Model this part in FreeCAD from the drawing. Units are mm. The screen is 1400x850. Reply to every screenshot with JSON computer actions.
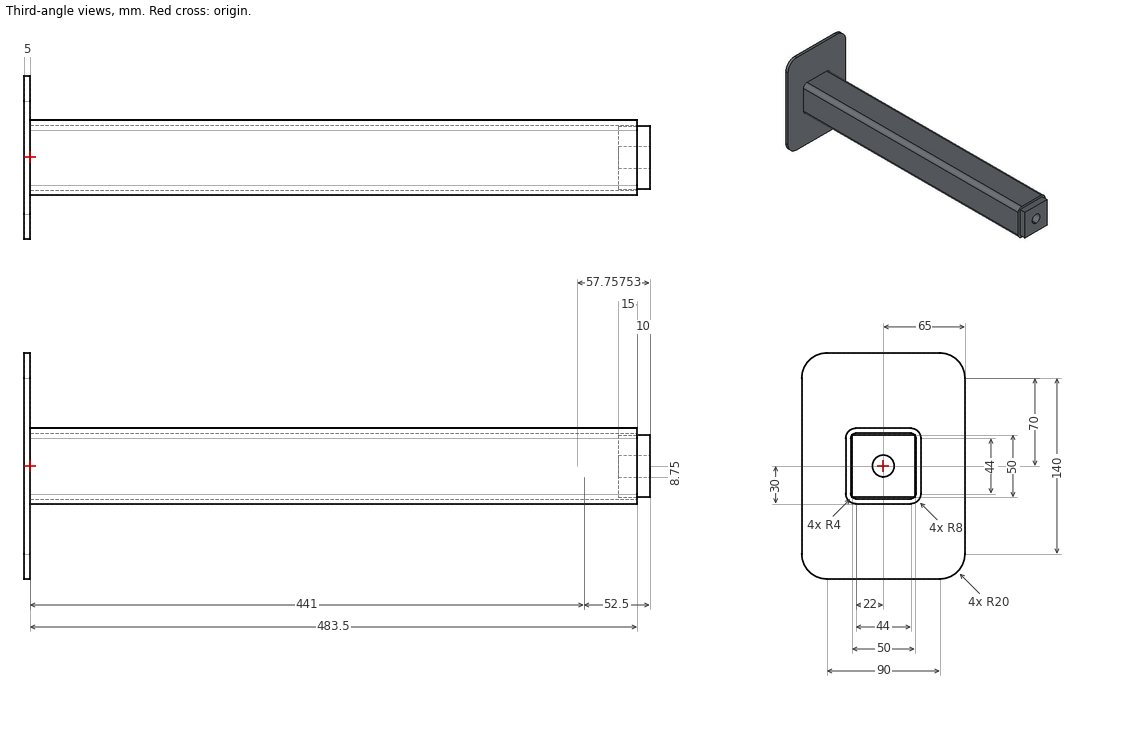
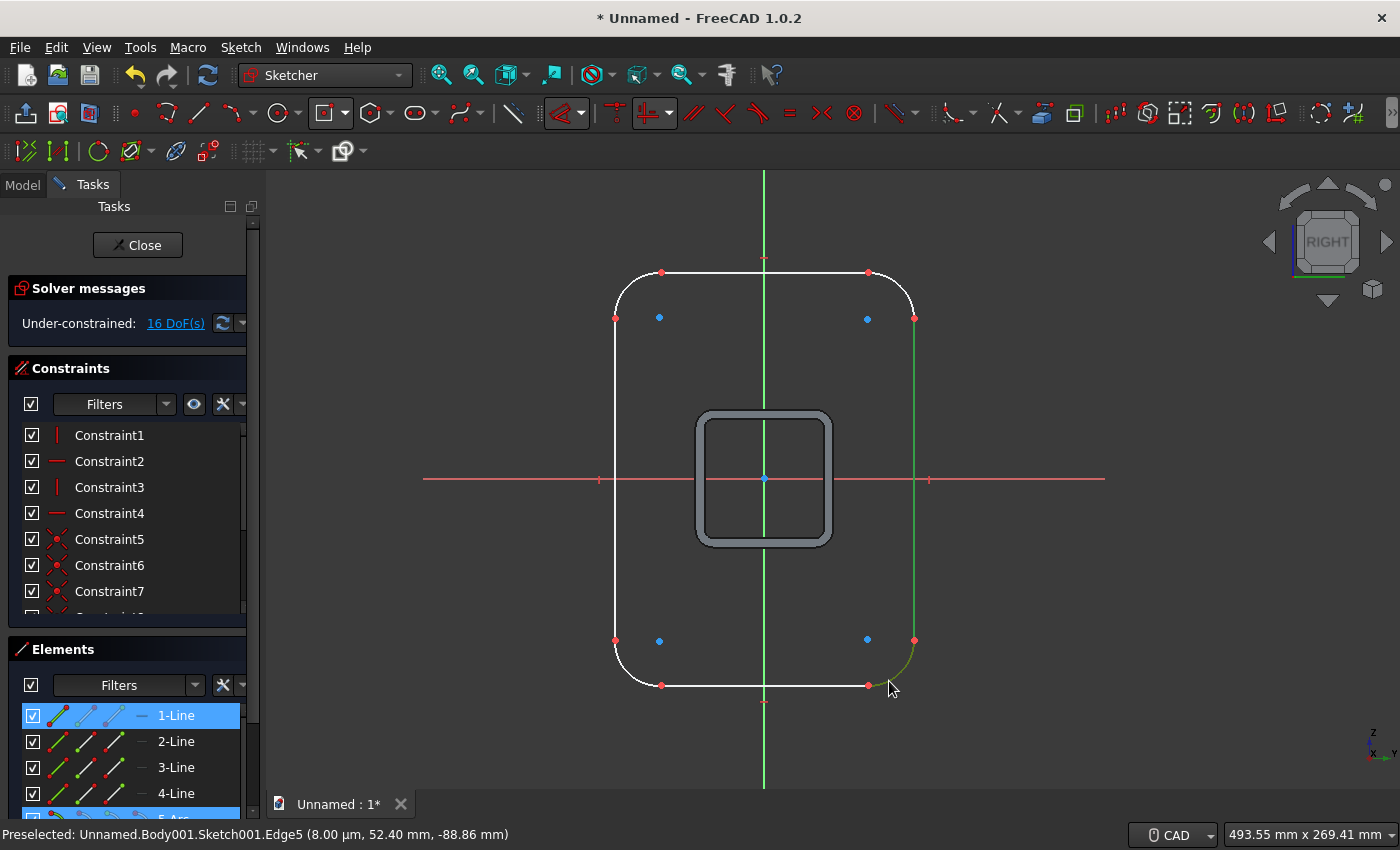
{"action": "left_click", "coordinate": [758, 114]}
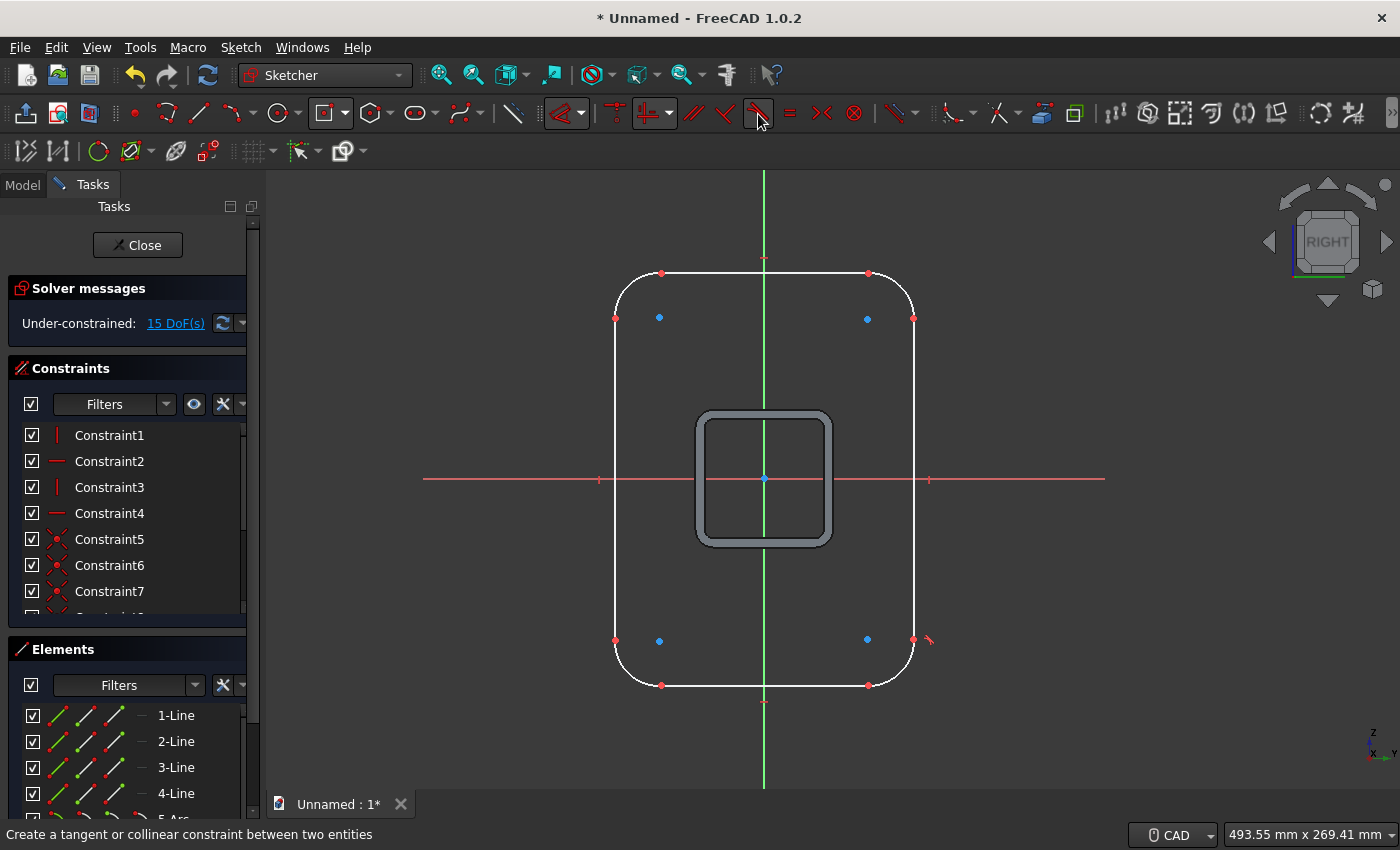
{"action": "left_click", "coordinate": [914, 415]}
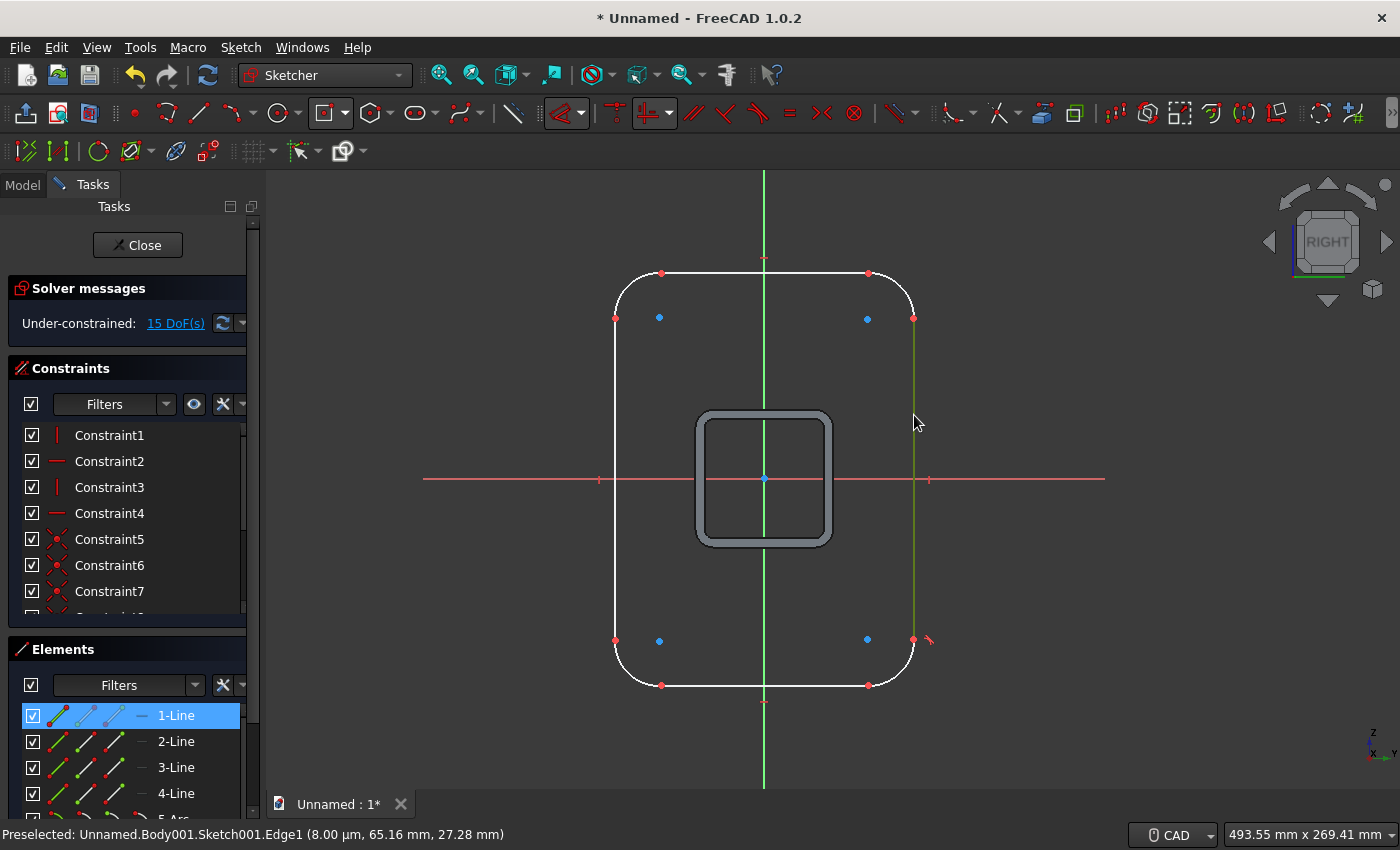
{"action": "left_click", "coordinate": [909, 298]}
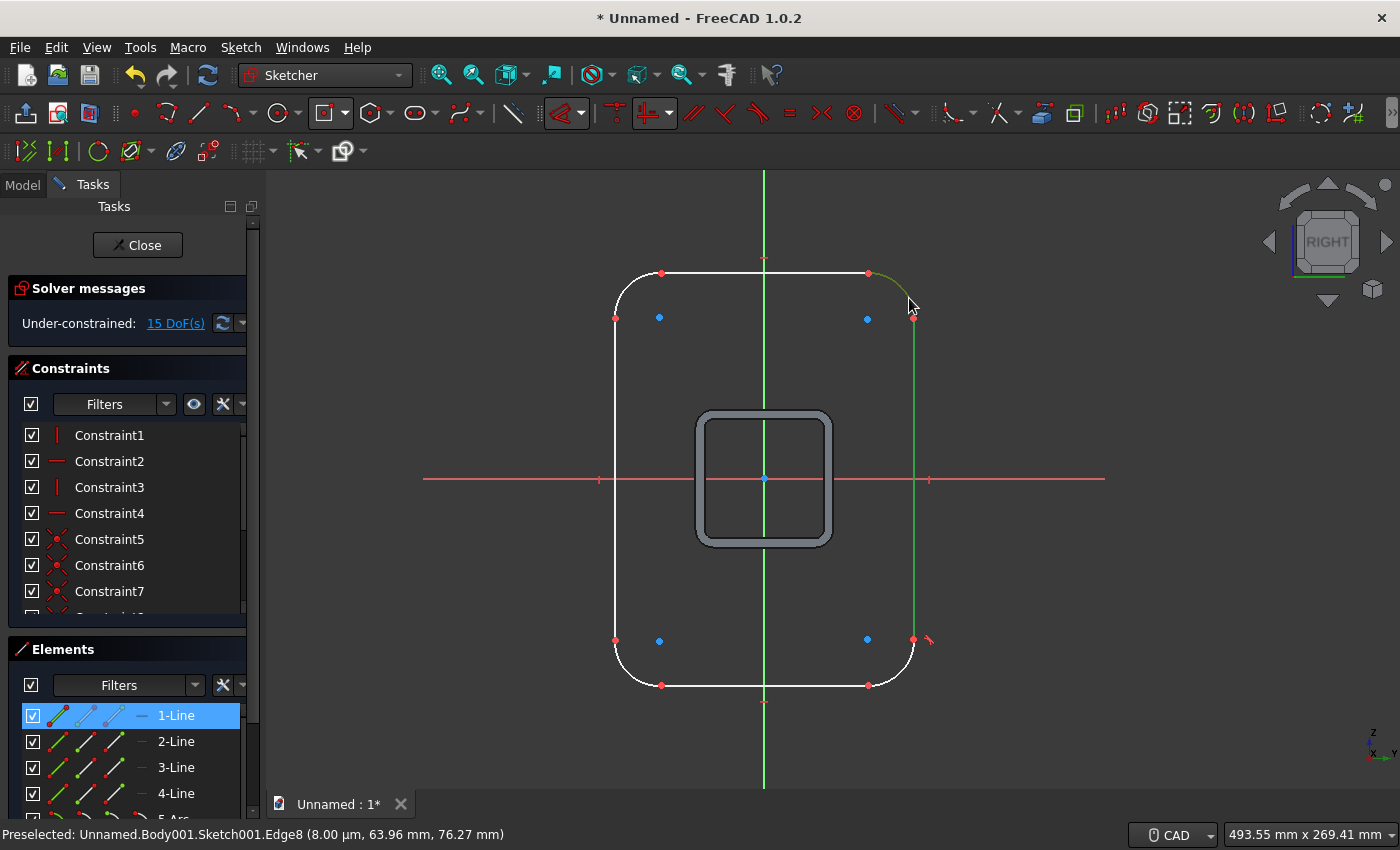
{"action": "left_click", "coordinate": [758, 114]}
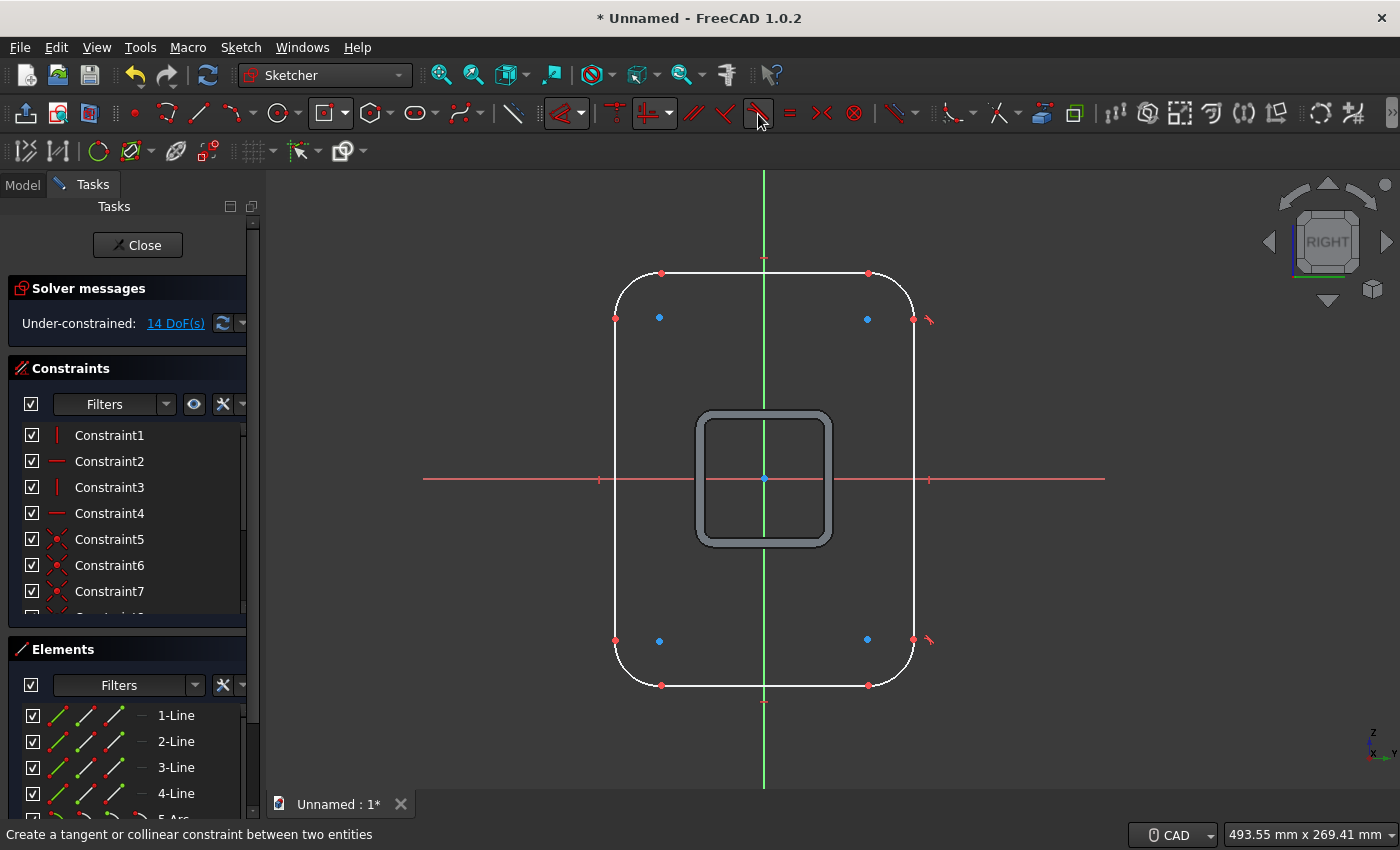
{"action": "left_click", "coordinate": [806, 686]}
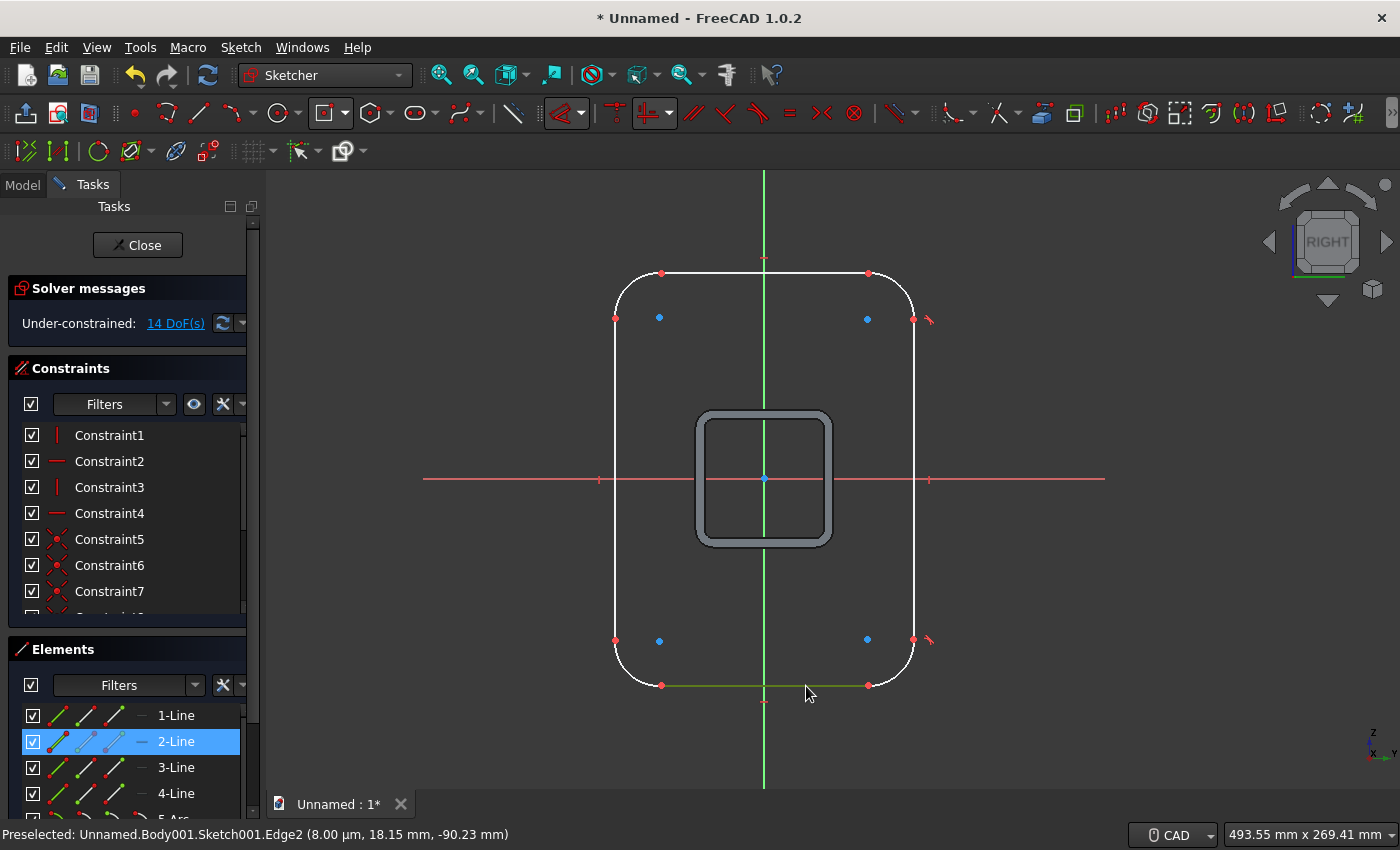
{"action": "left_click", "coordinate": [889, 681]}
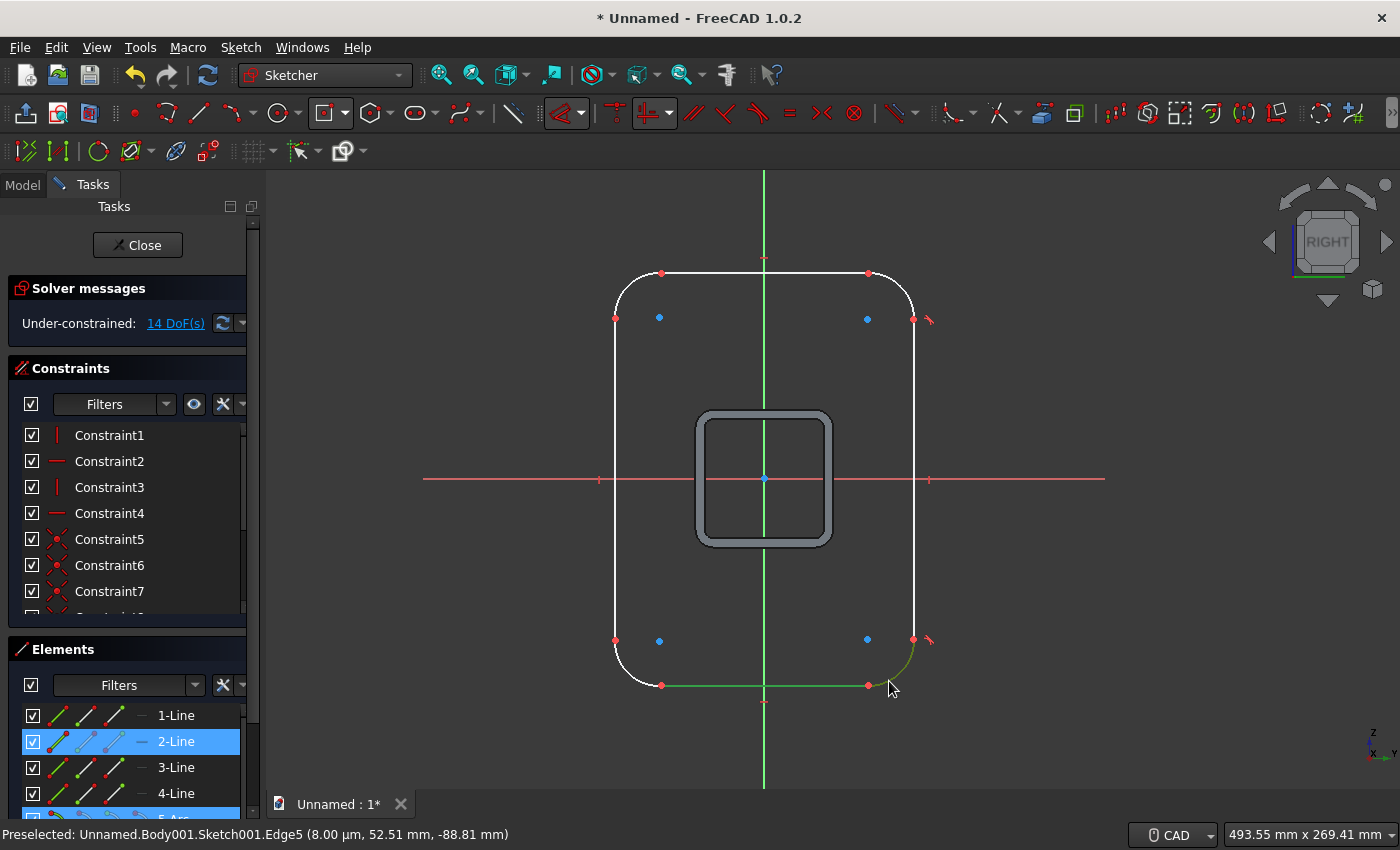
{"action": "left_click", "coordinate": [758, 114]}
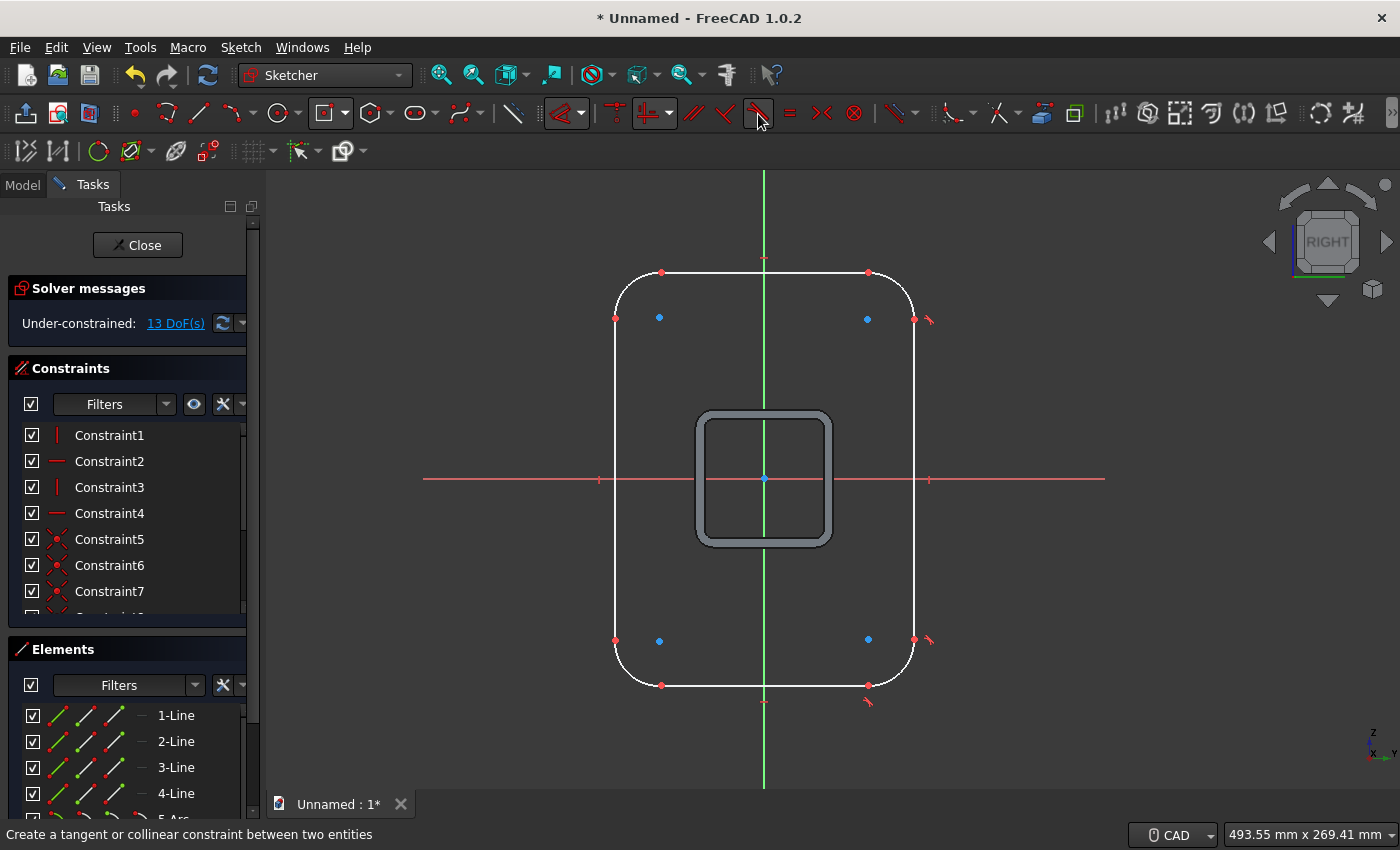
{"action": "left_click", "coordinate": [806, 686]}